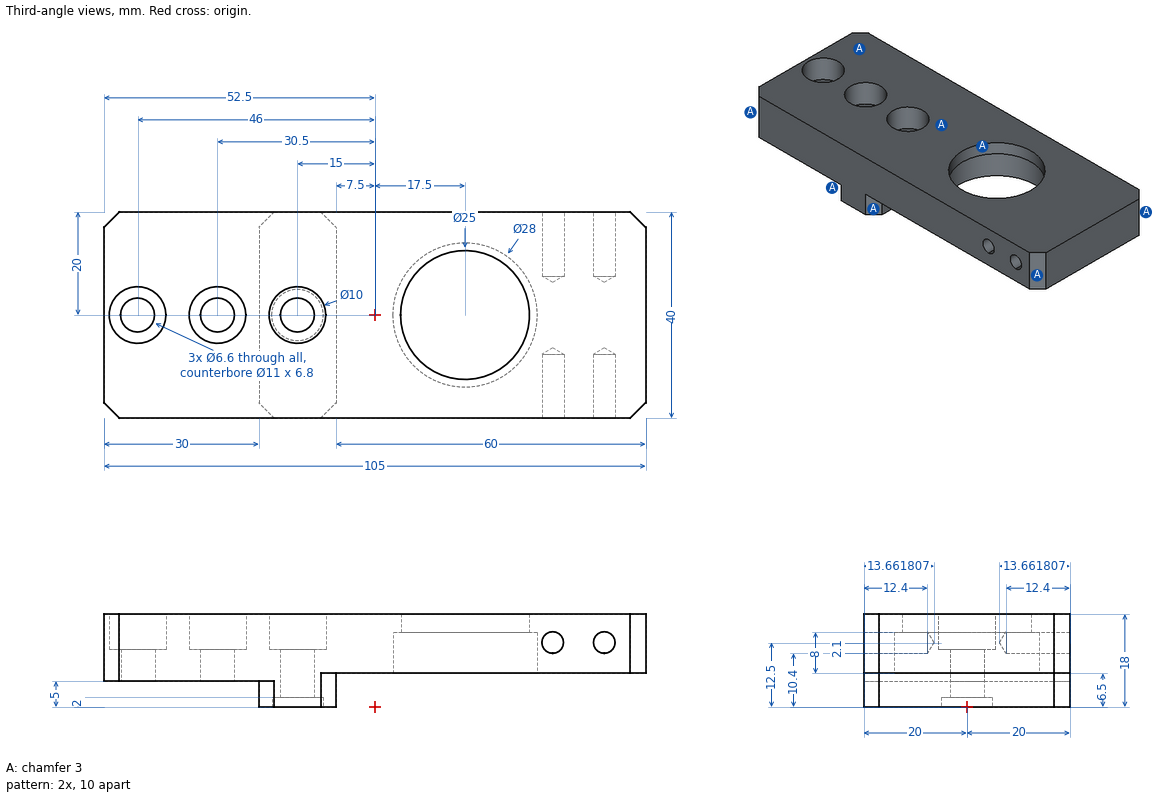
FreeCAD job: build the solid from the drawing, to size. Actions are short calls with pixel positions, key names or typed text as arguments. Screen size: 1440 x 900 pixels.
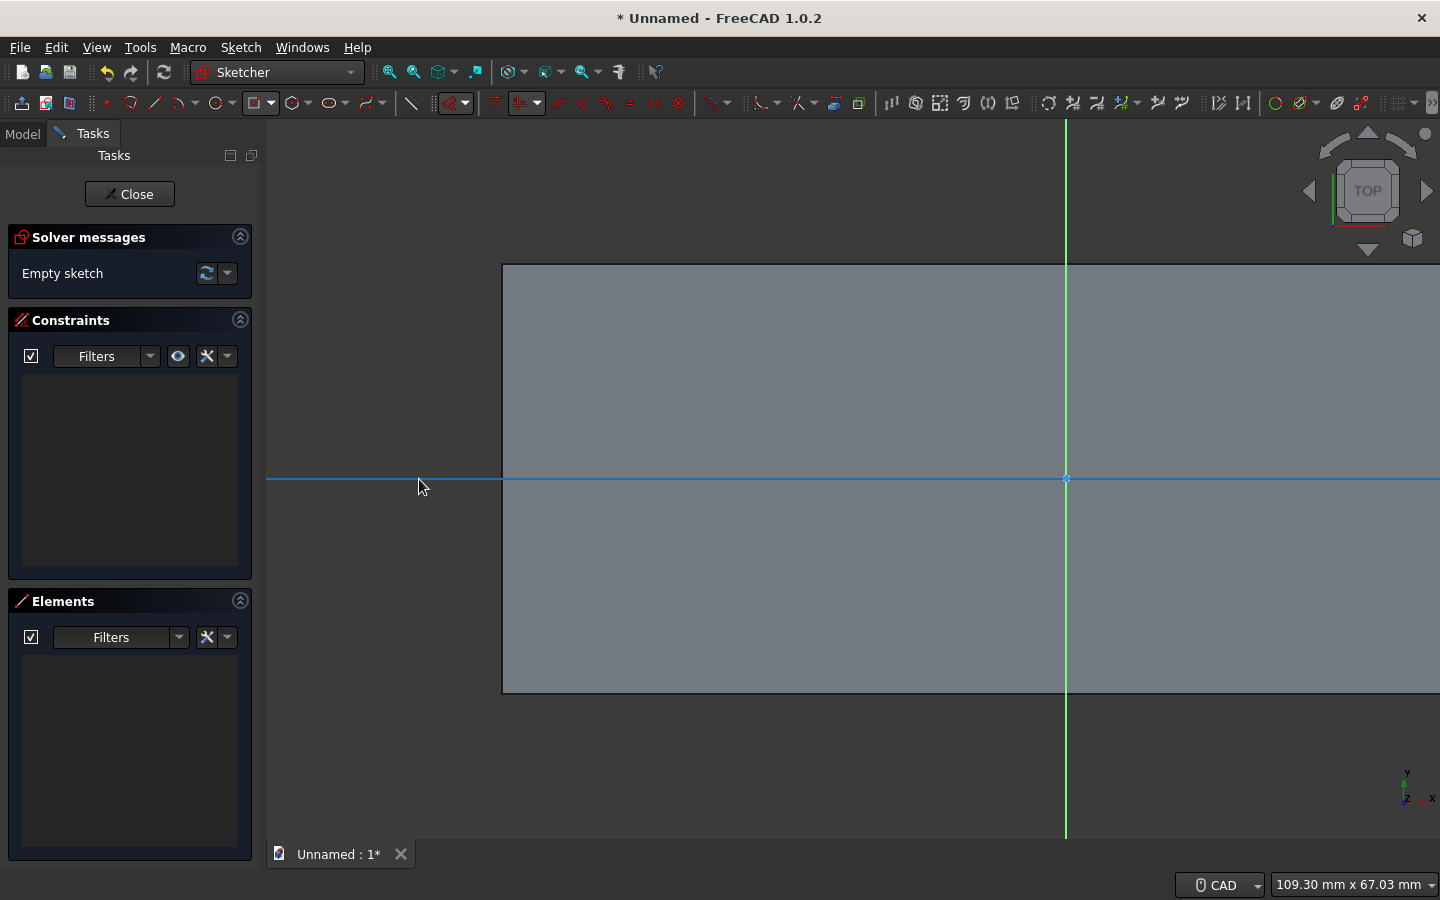
key(g)
key(r)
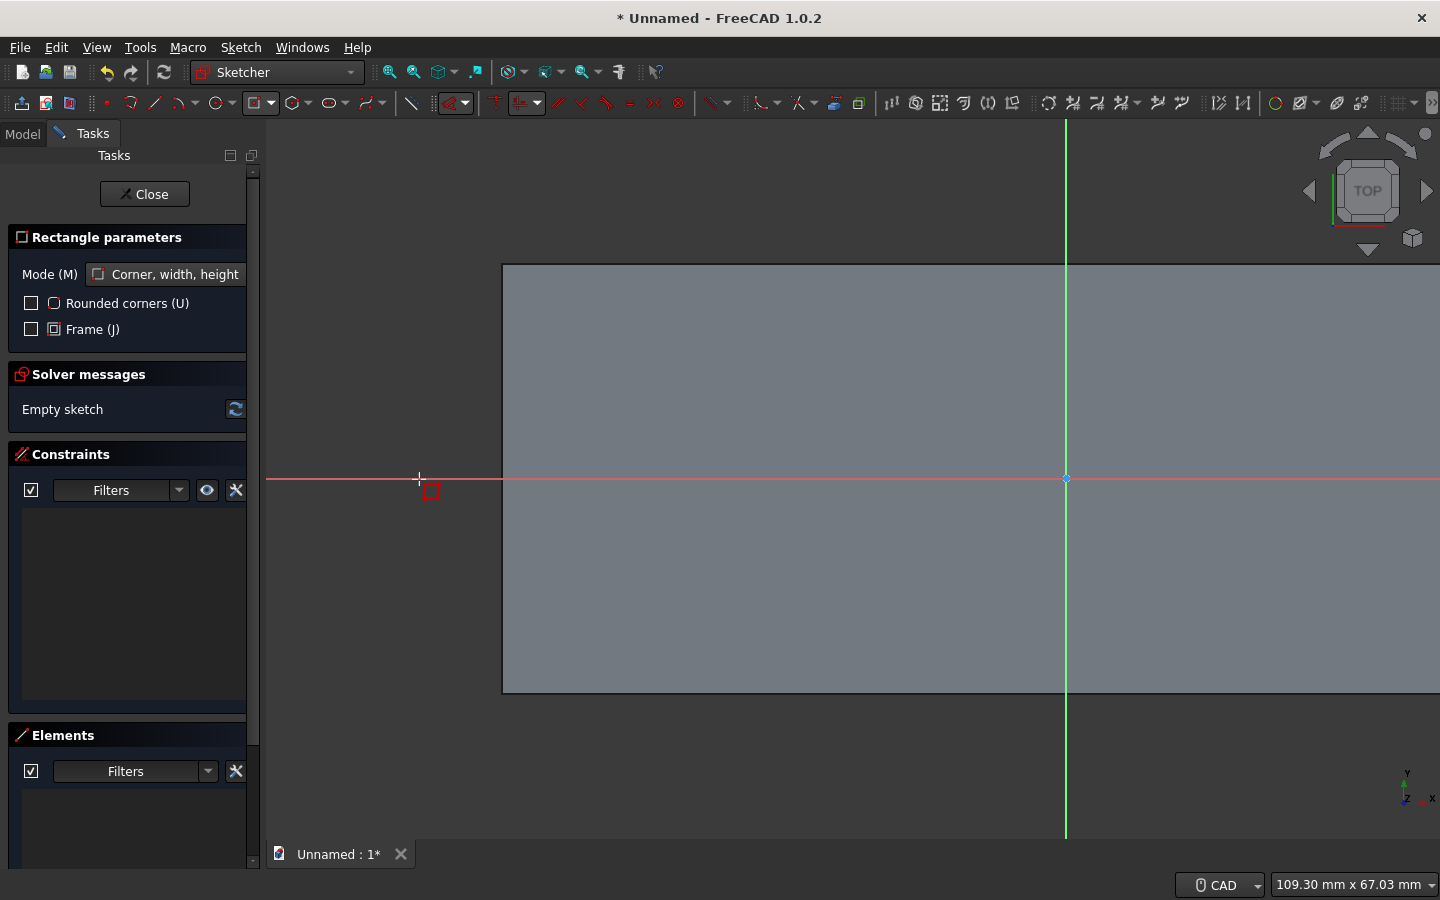
click(502, 264)
click(825, 694)
key(Escape)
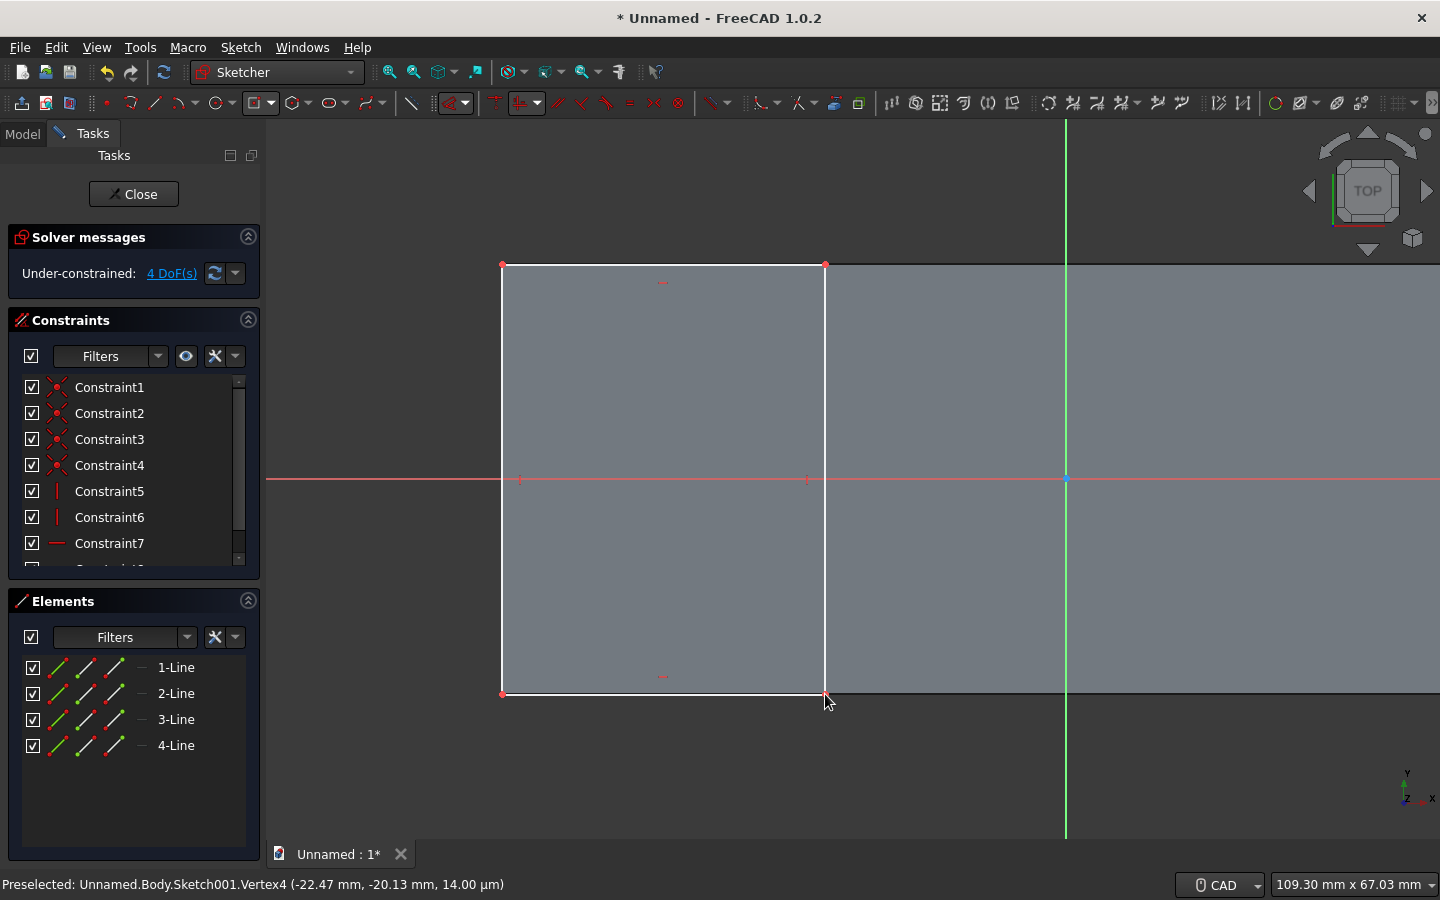
click(502, 394)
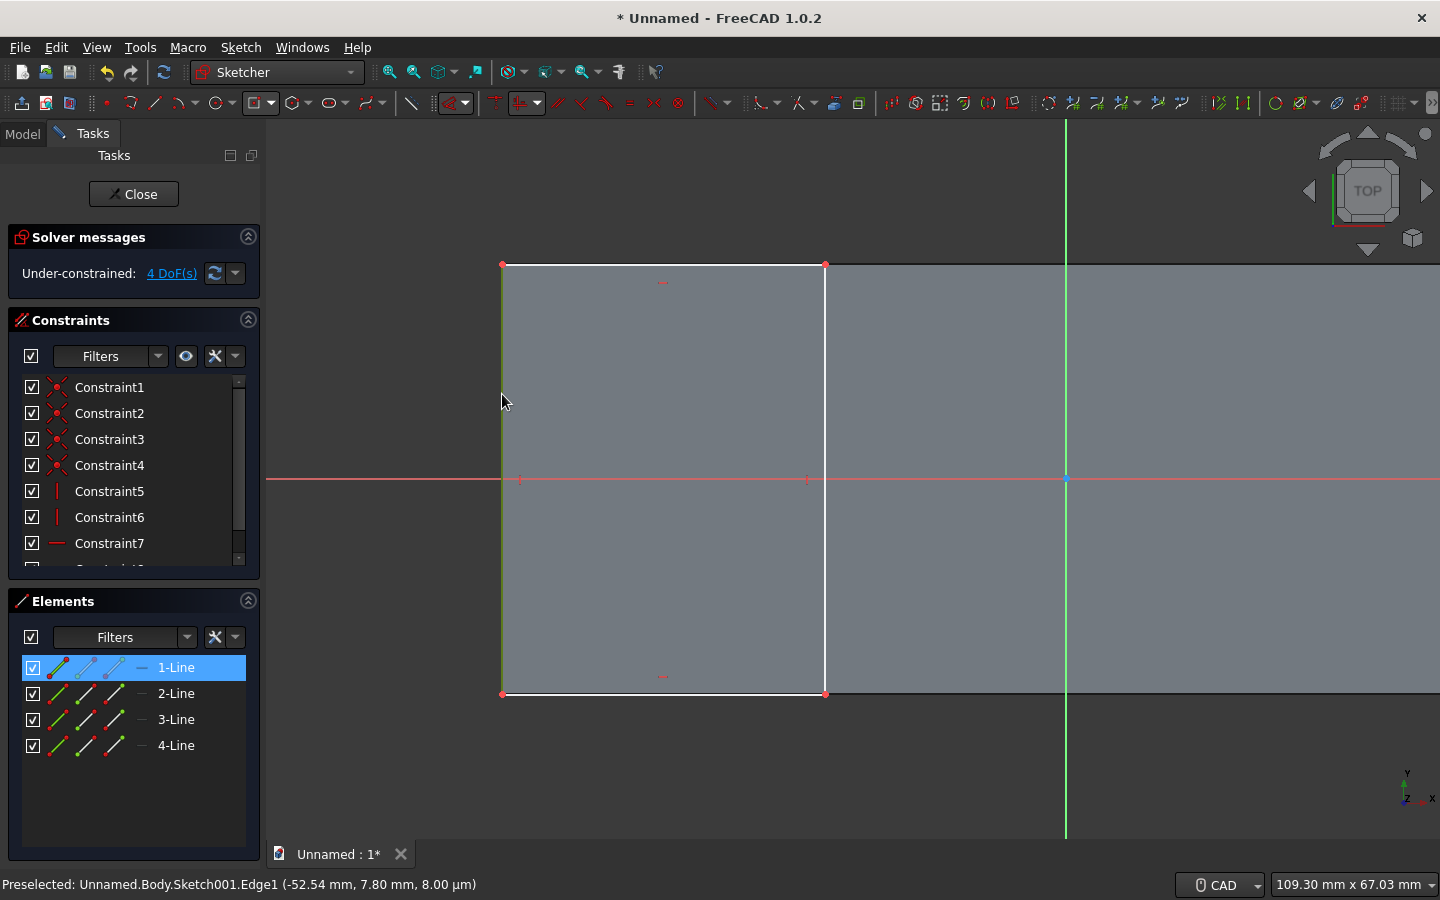
key(i)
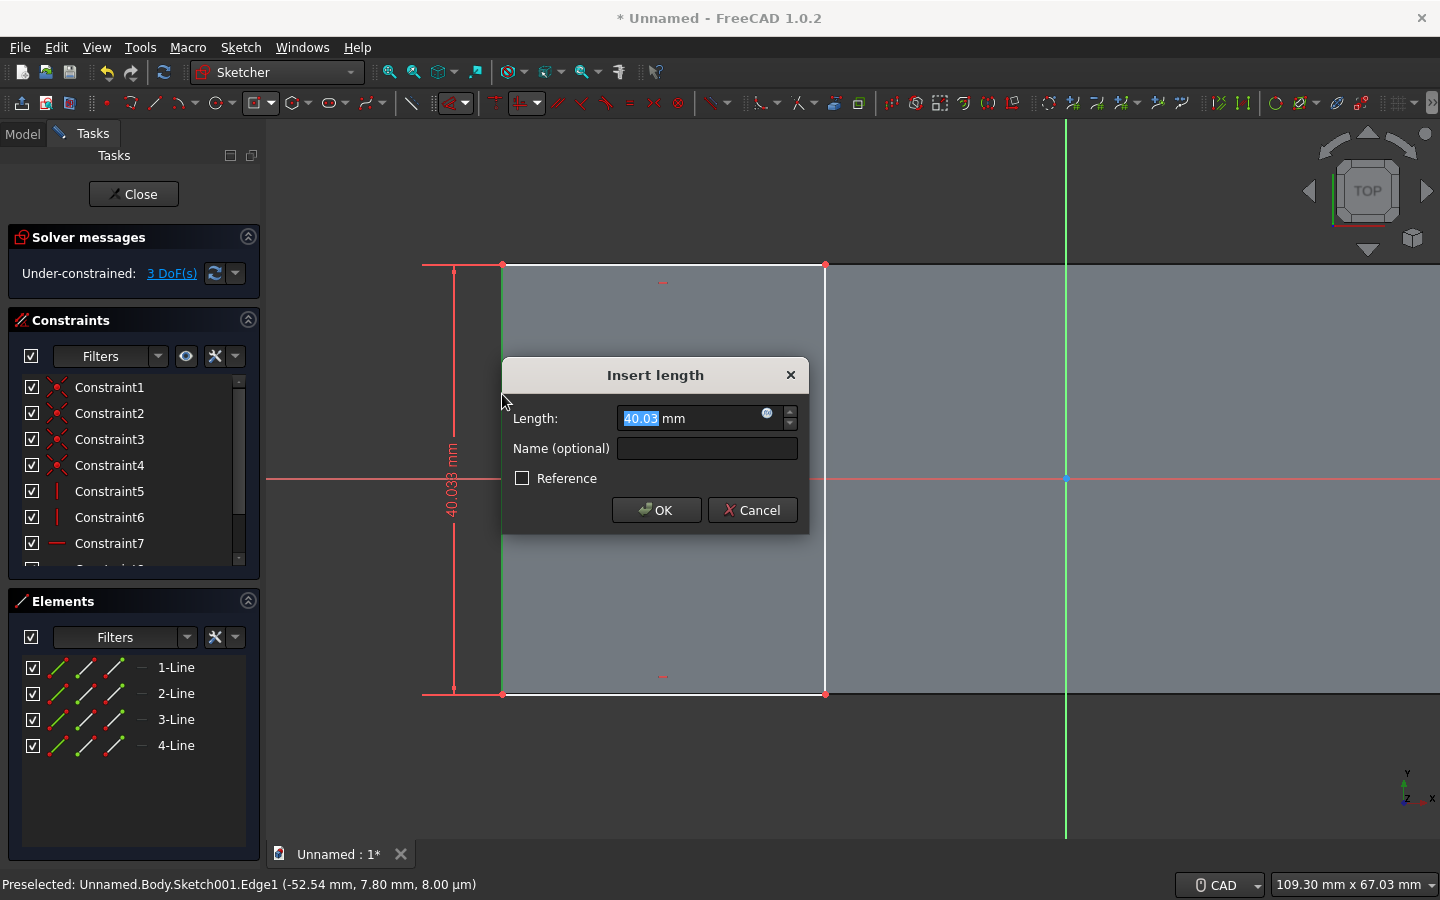
text(40)
key(Return)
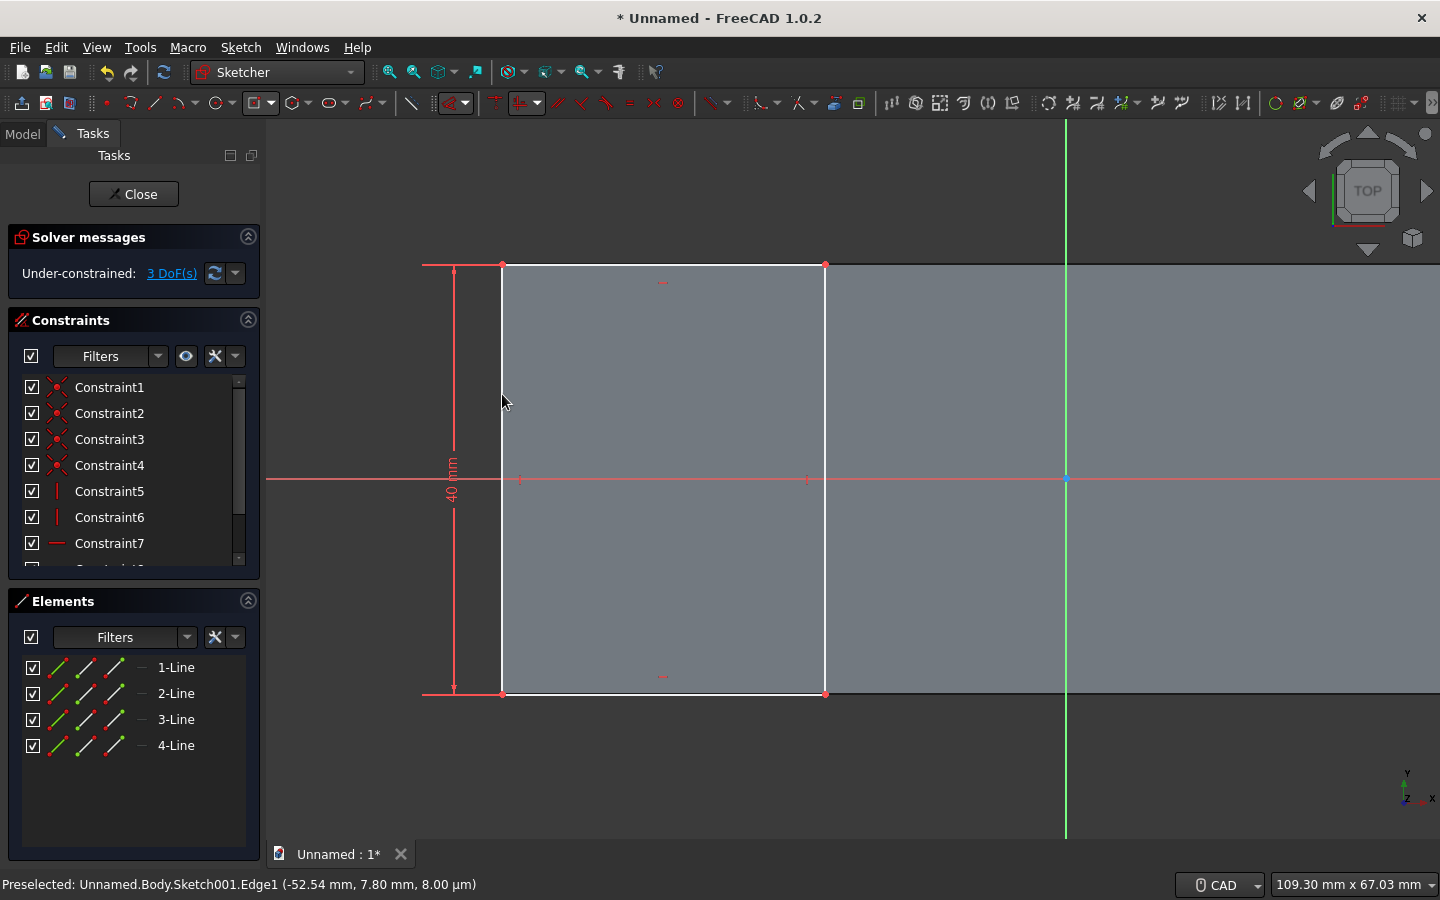
click(599, 695)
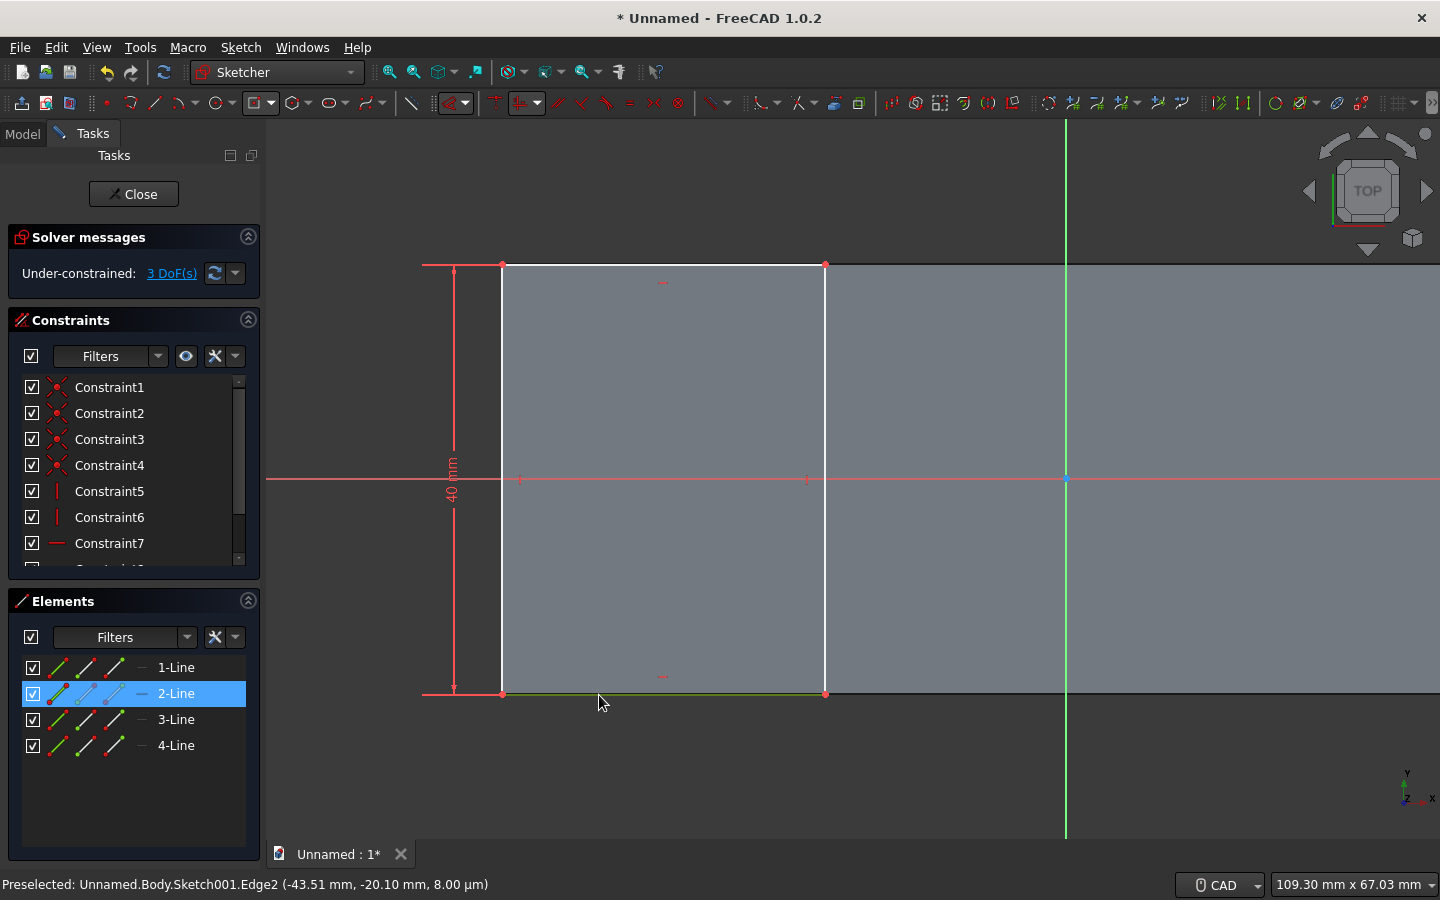
key(l)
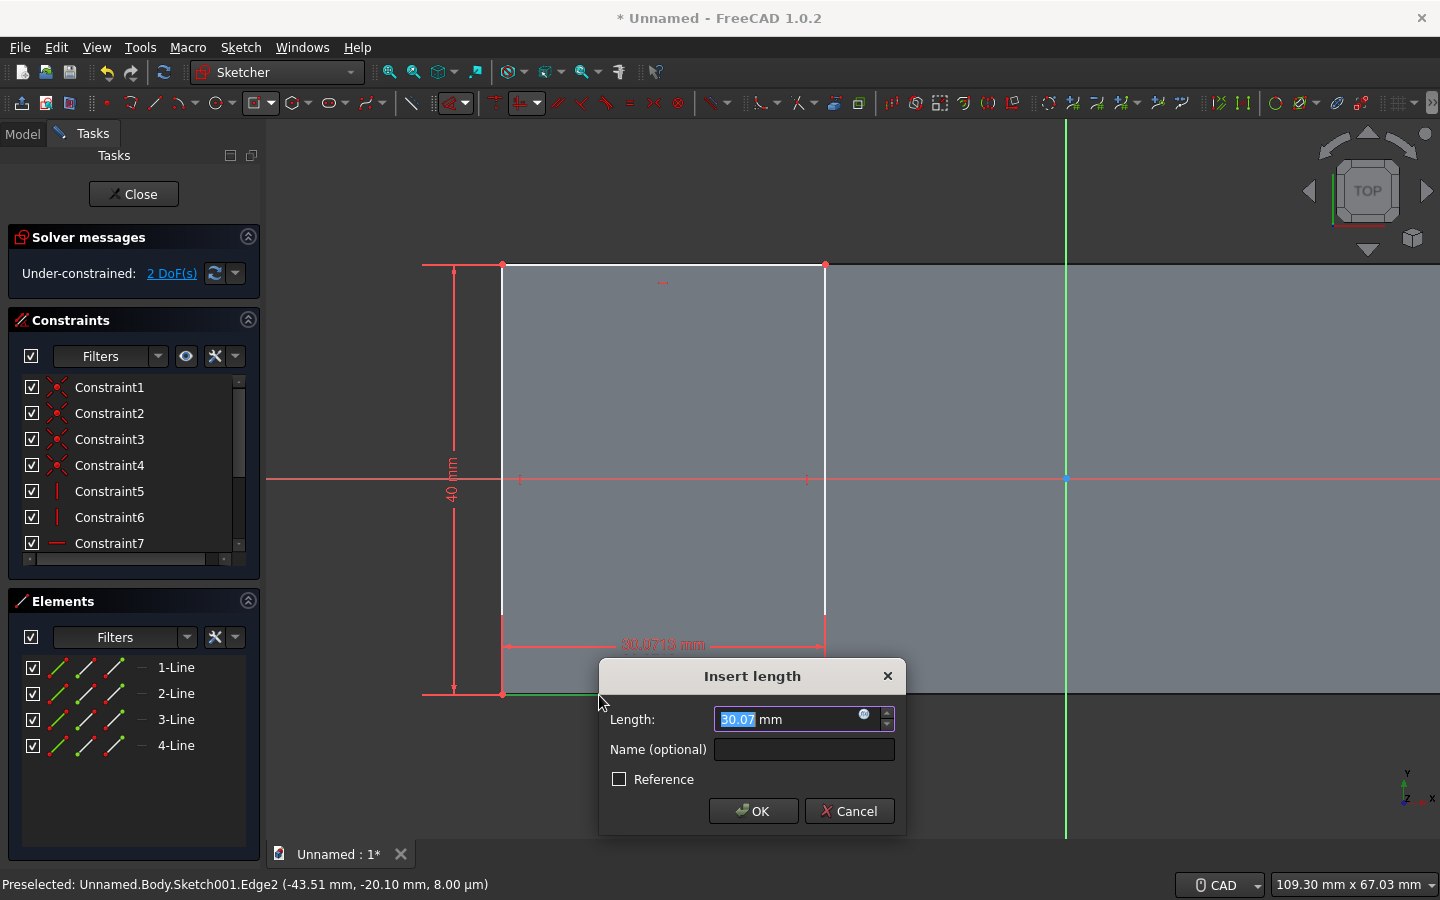
text(30)
key(Return)